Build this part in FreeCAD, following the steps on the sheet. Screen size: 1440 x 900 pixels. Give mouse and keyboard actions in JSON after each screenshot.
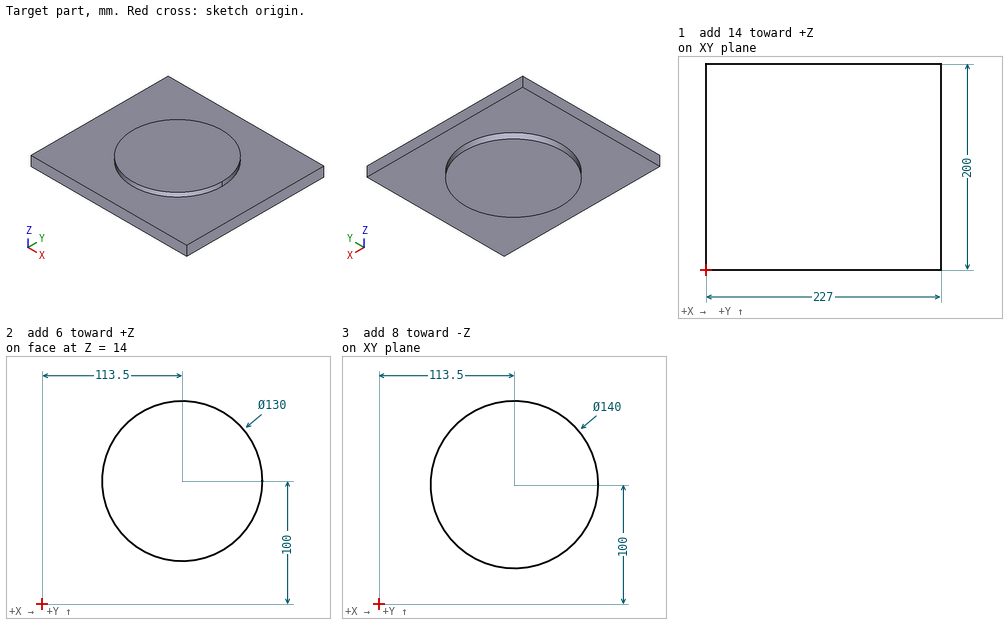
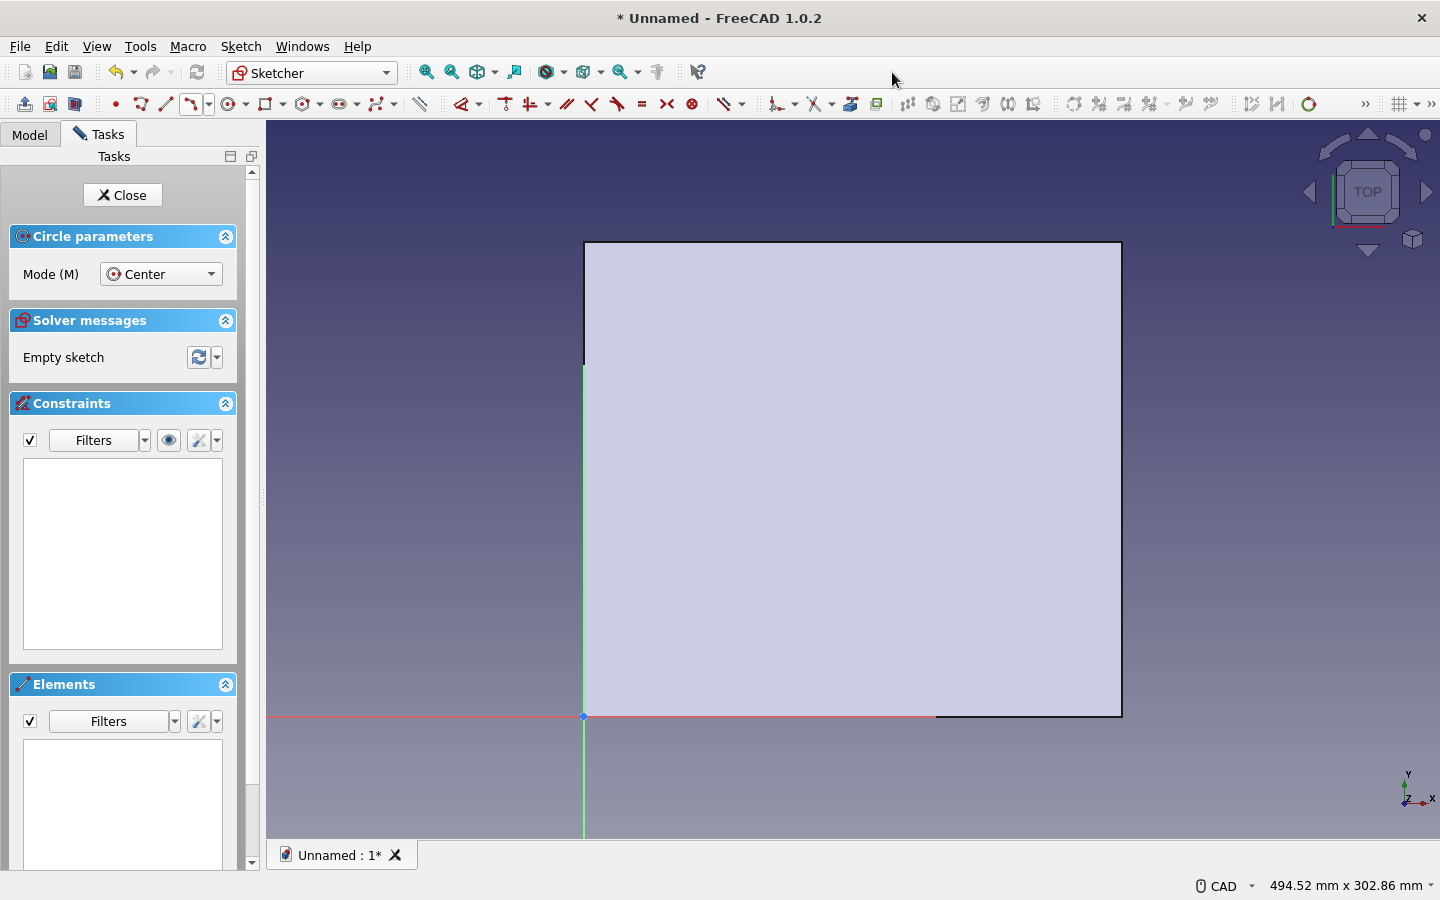
{"action": "left_click", "coordinate": [853, 480]}
{"action": "mouse_move", "coordinate": [962, 370]}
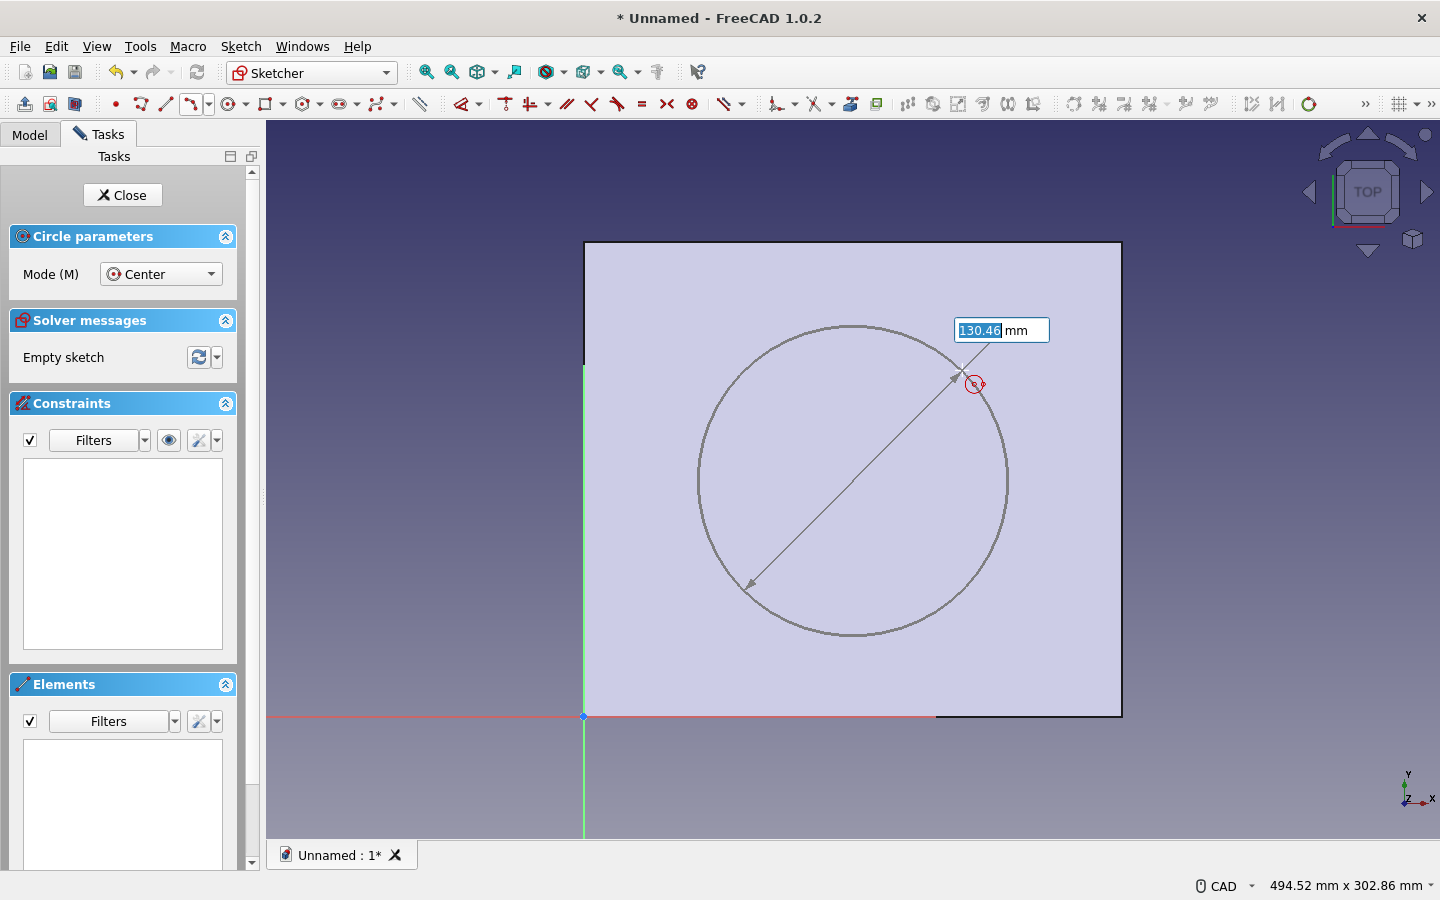
{"action": "type", "text": "130"}
{"action": "key", "text": "Return"}
{"action": "key", "text": "Escape"}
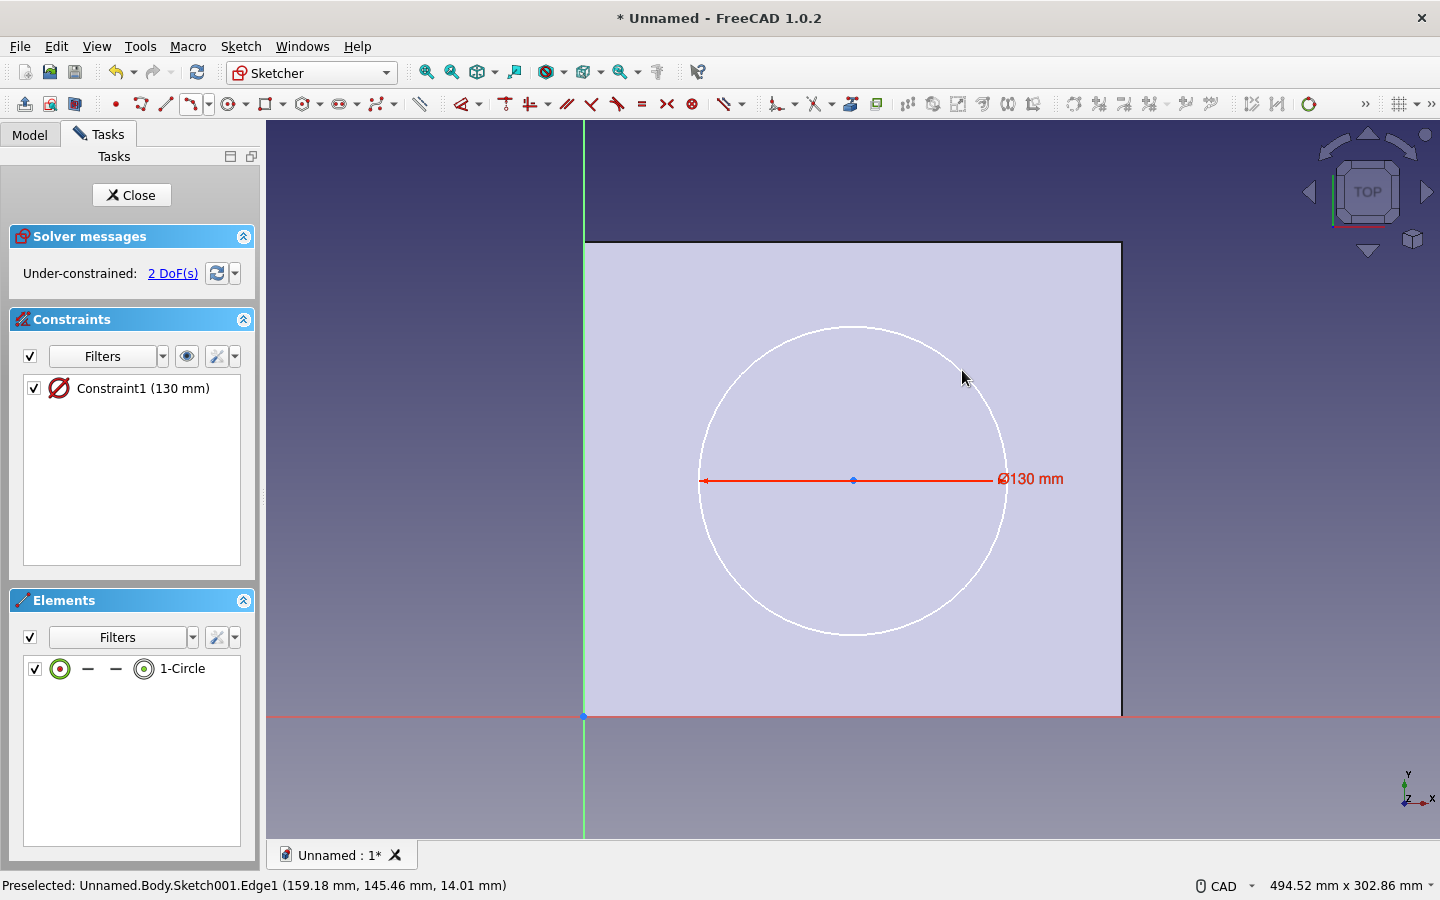
{"action": "left_click", "coordinate": [853, 481]}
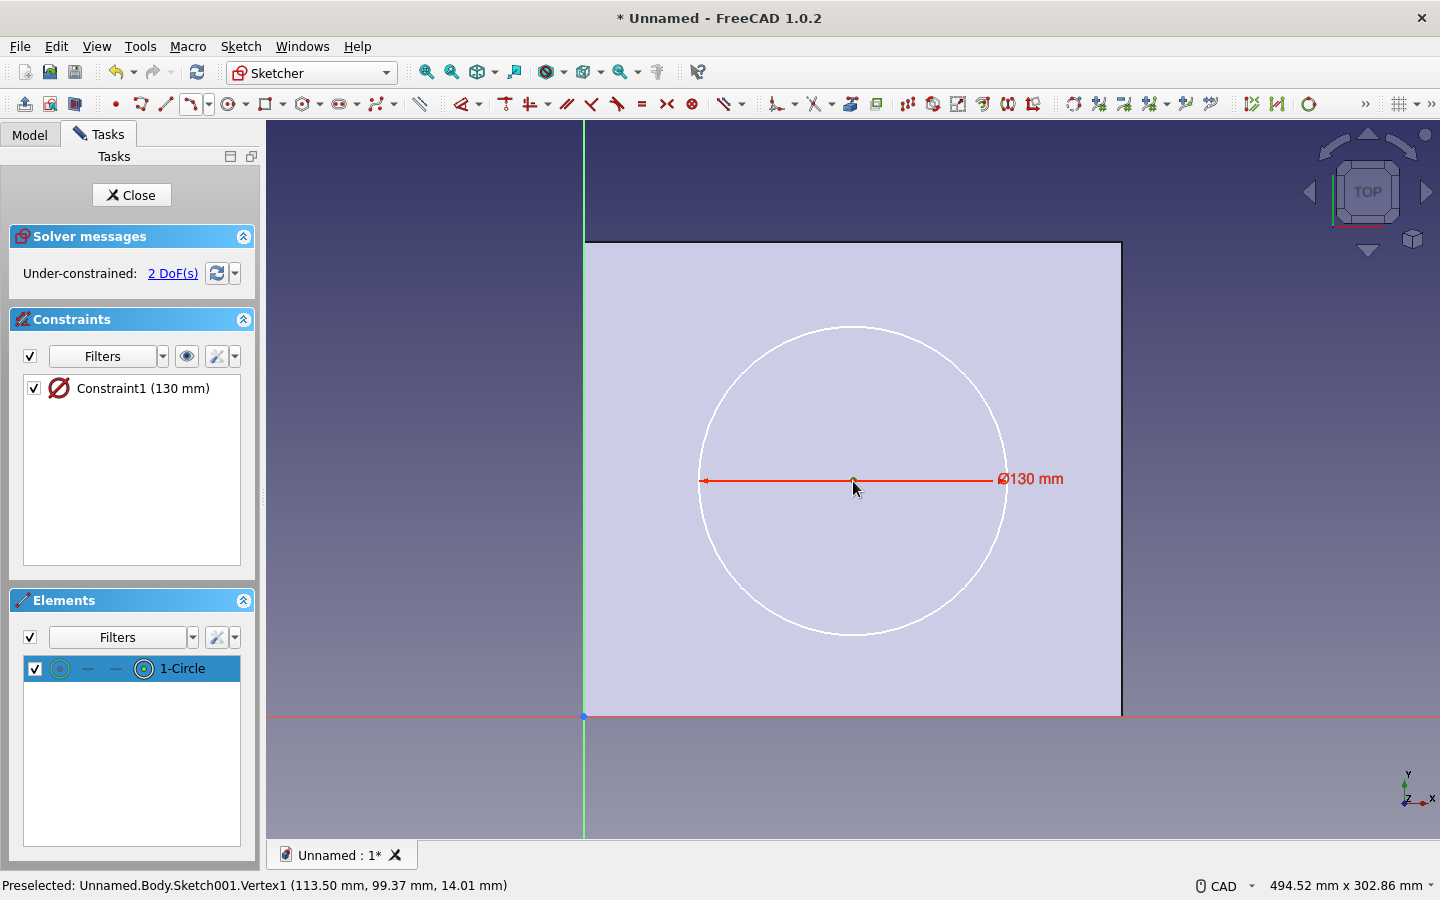
{"action": "key", "text": "i"}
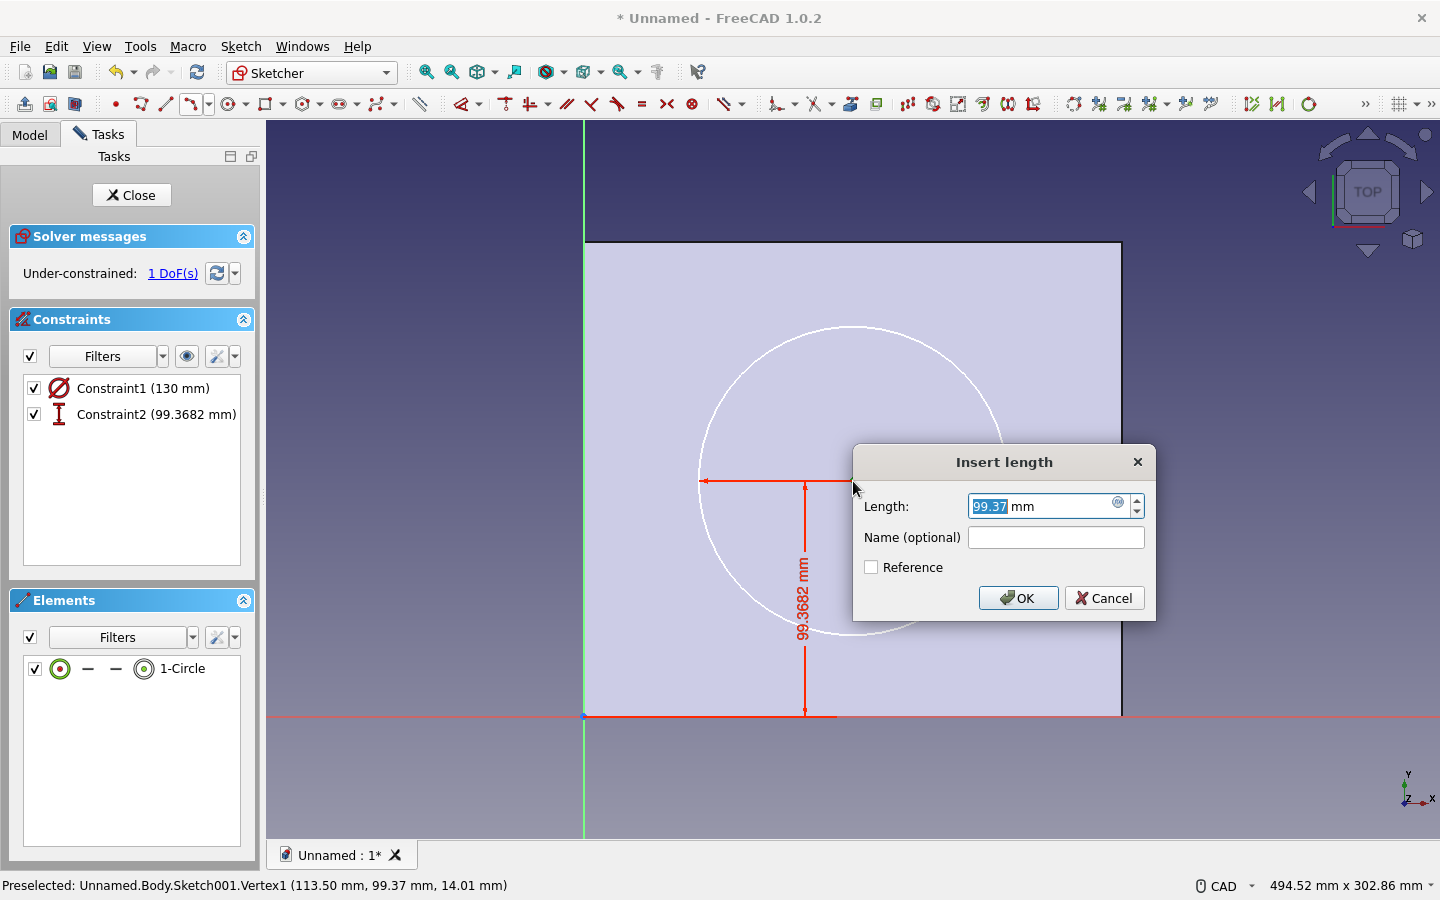
{"action": "type", "text": "100"}
{"action": "key", "text": "Return"}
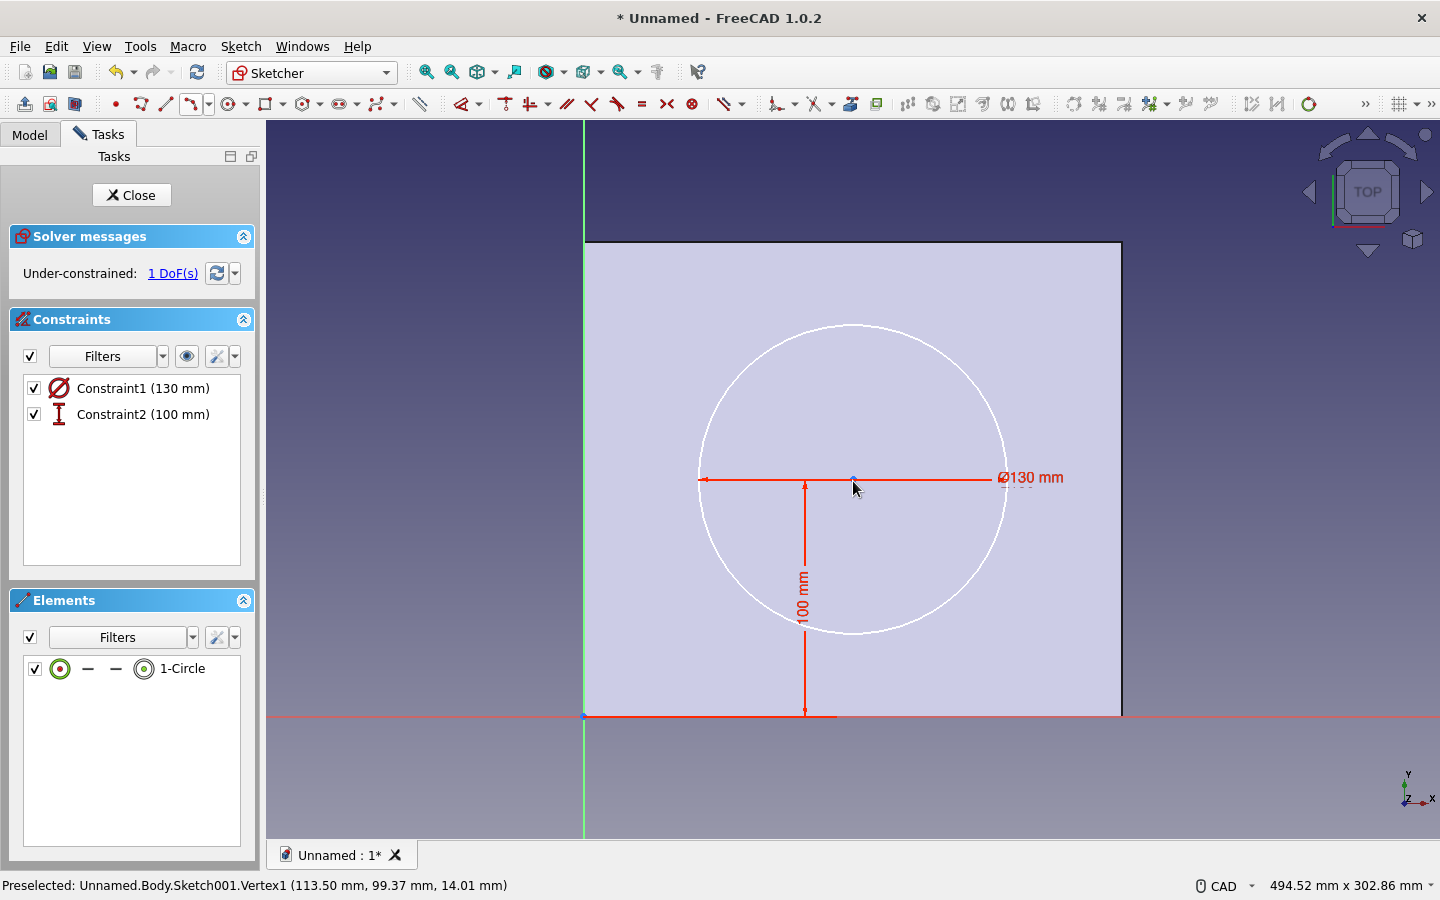
{"action": "left_click", "coordinate": [853, 480]}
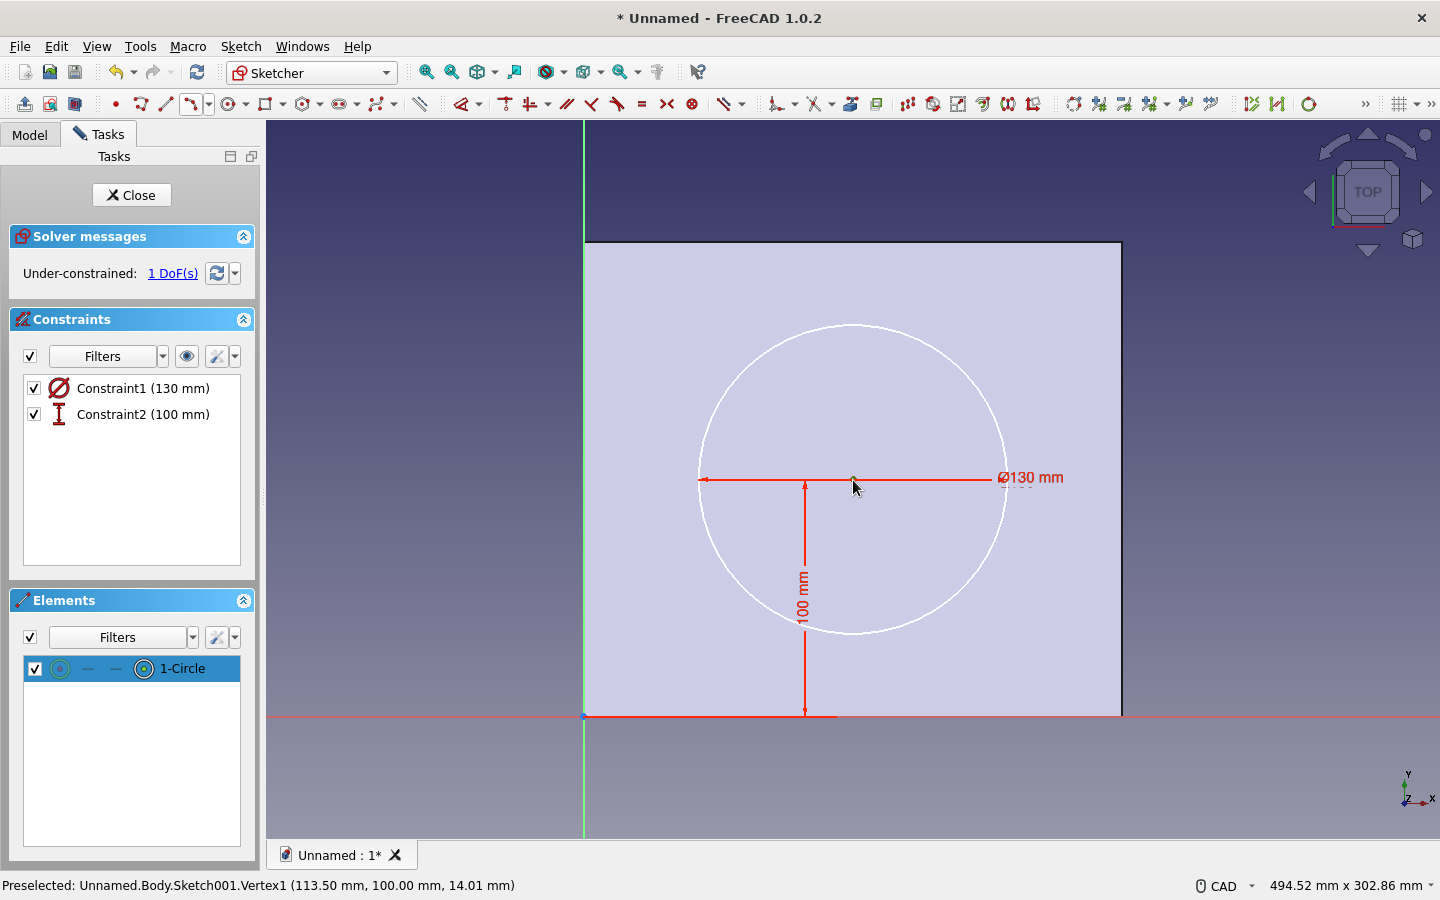
{"action": "key", "text": "l"}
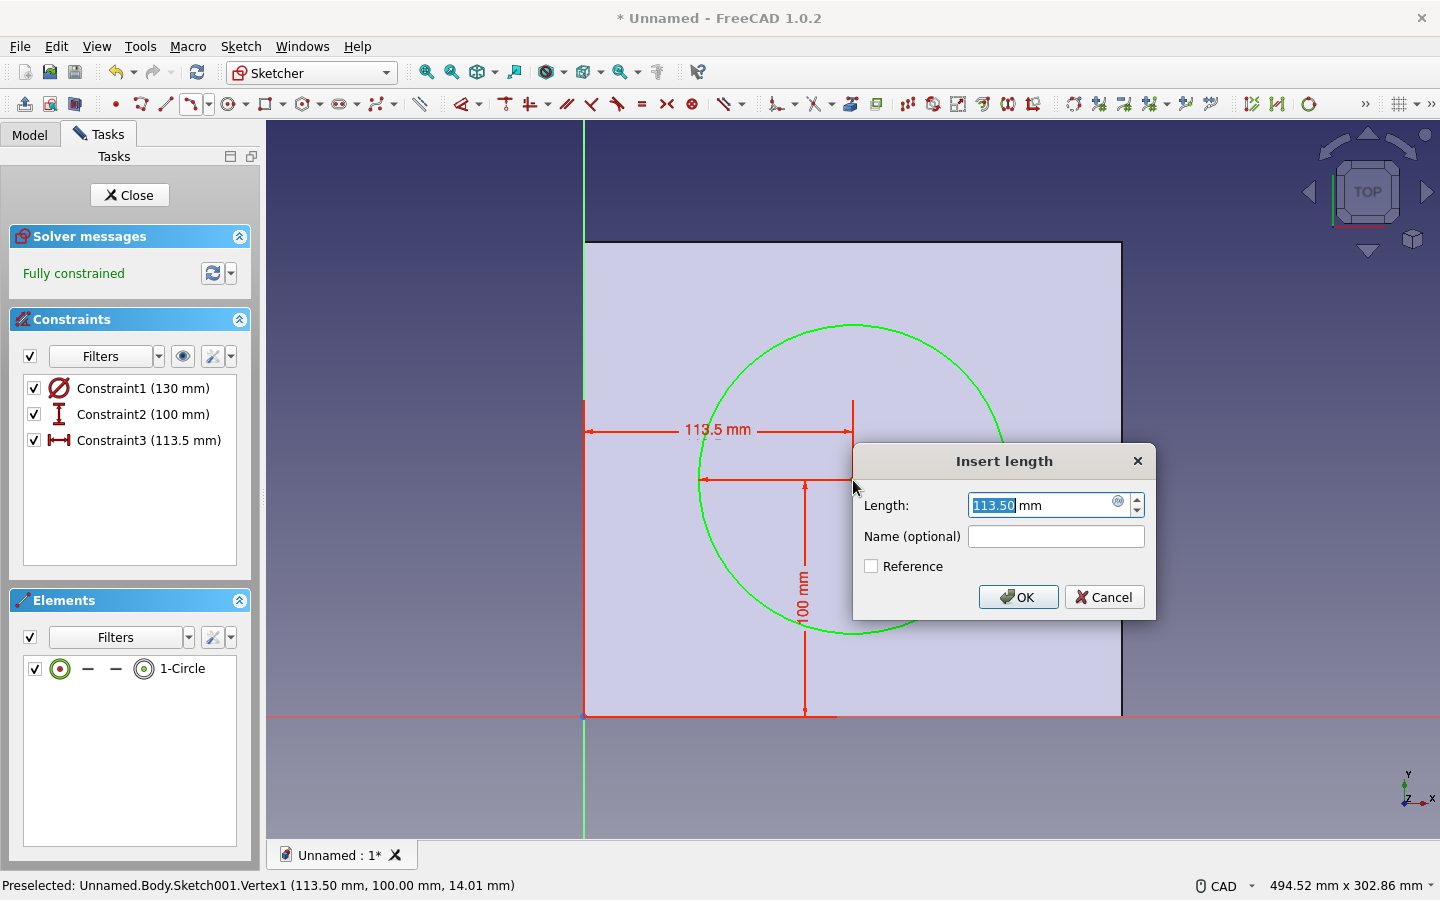
{"action": "type", "text": "113.5"}
{"action": "key", "text": "Return"}